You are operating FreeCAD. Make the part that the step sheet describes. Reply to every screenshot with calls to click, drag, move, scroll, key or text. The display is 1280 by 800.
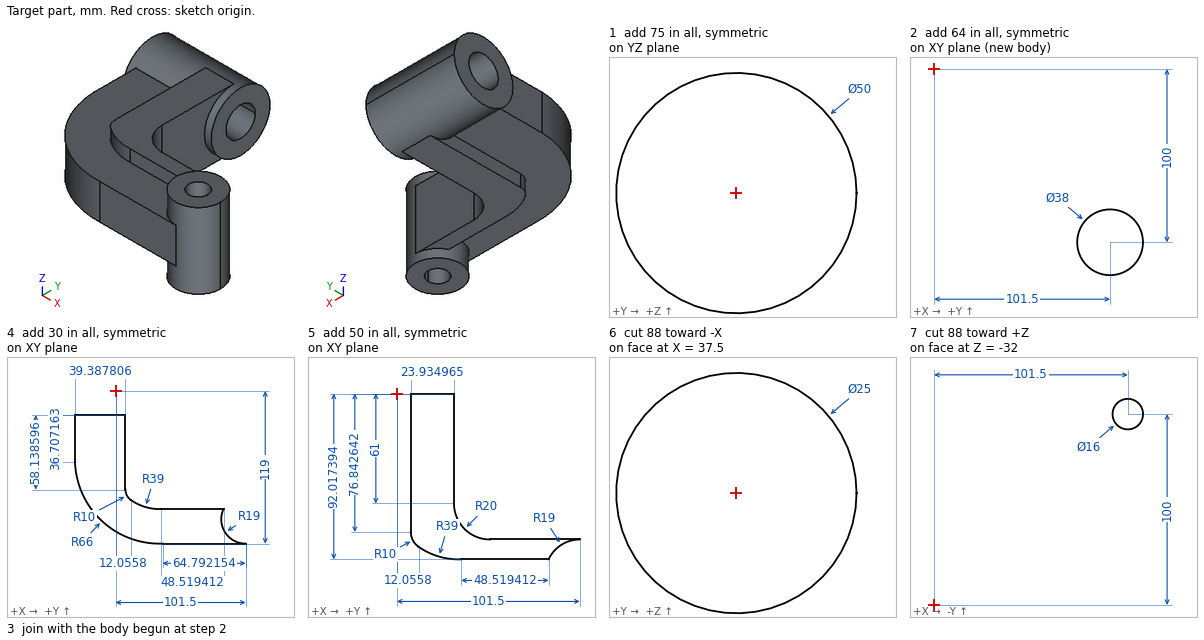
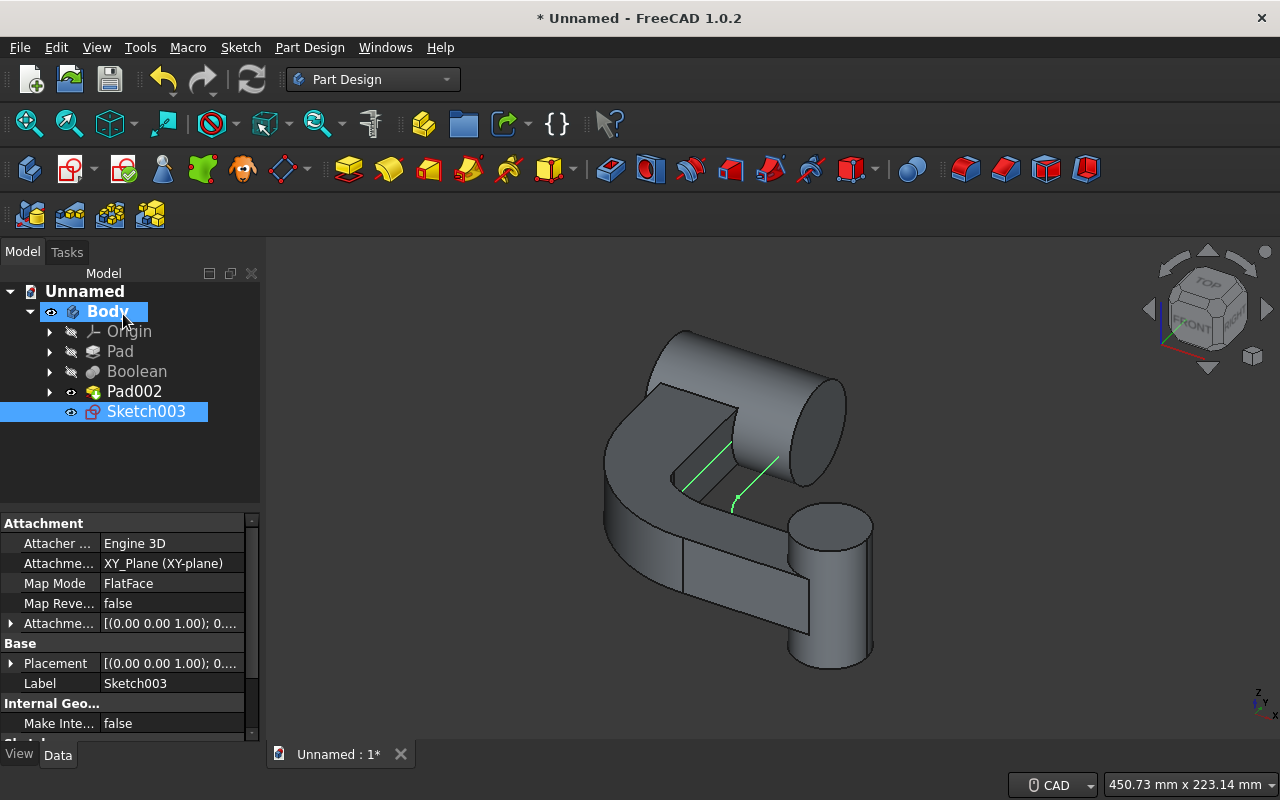
click(350, 170)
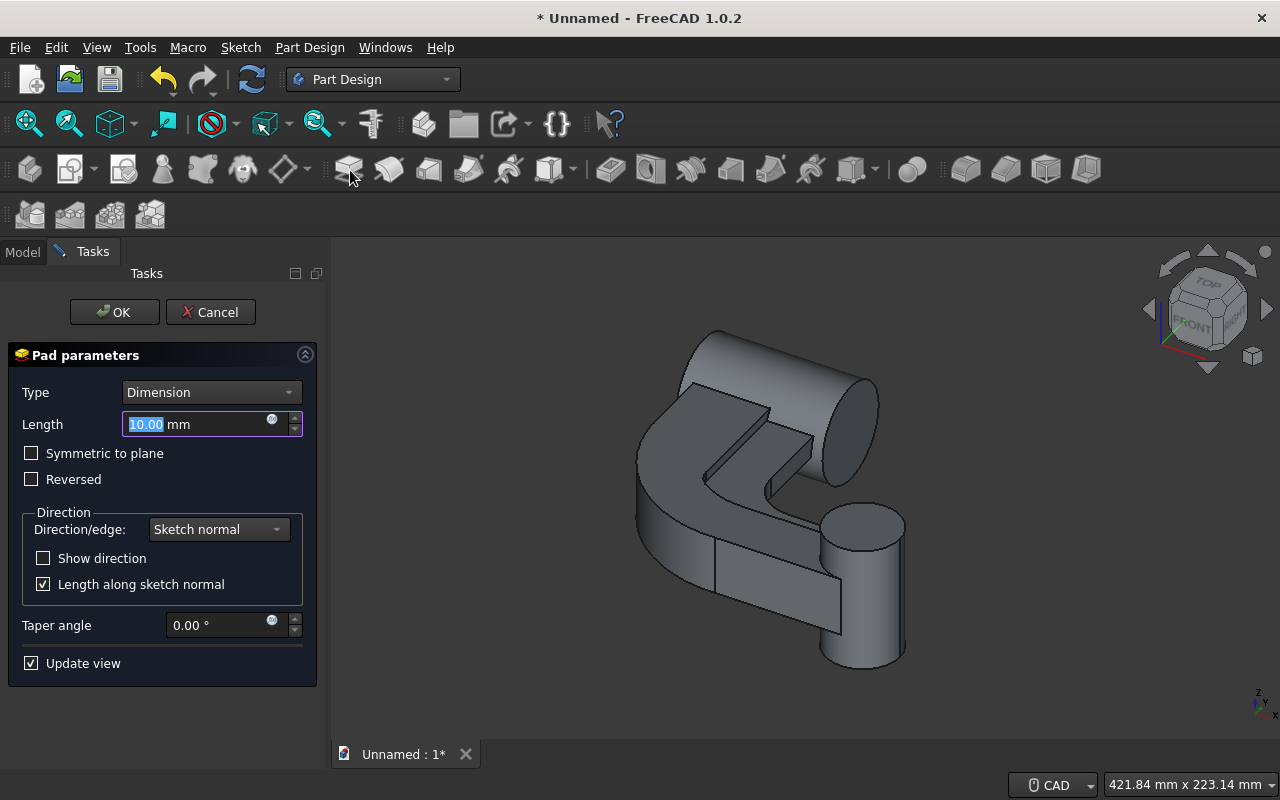
text(50)
key(Tab)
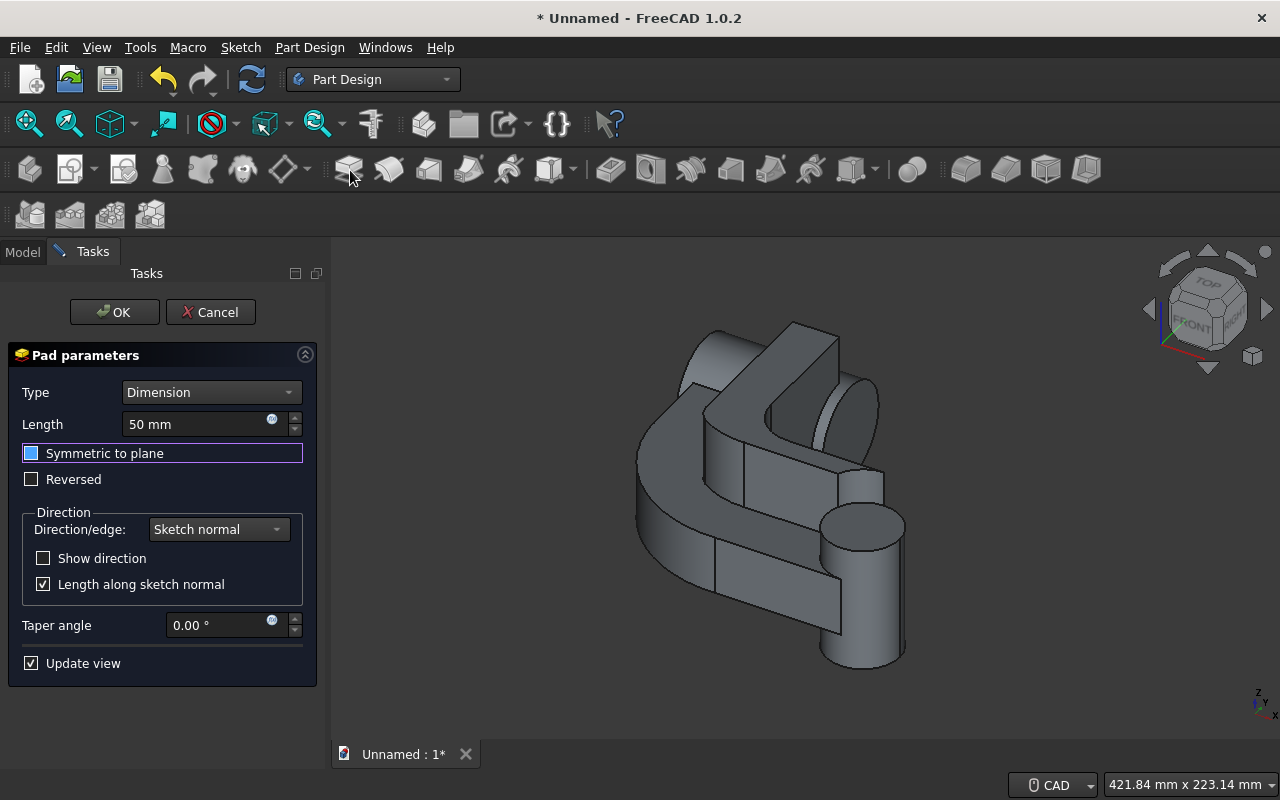
click(30, 453)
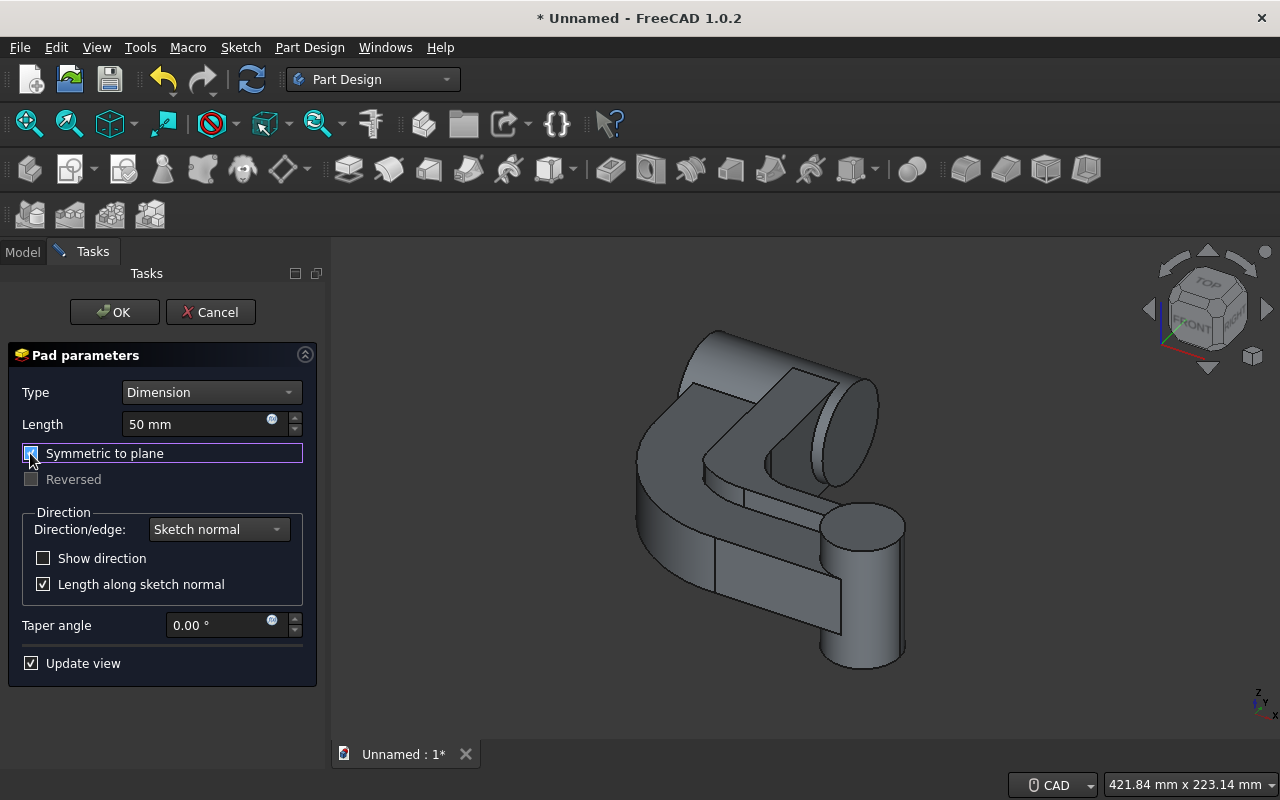
click(115, 312)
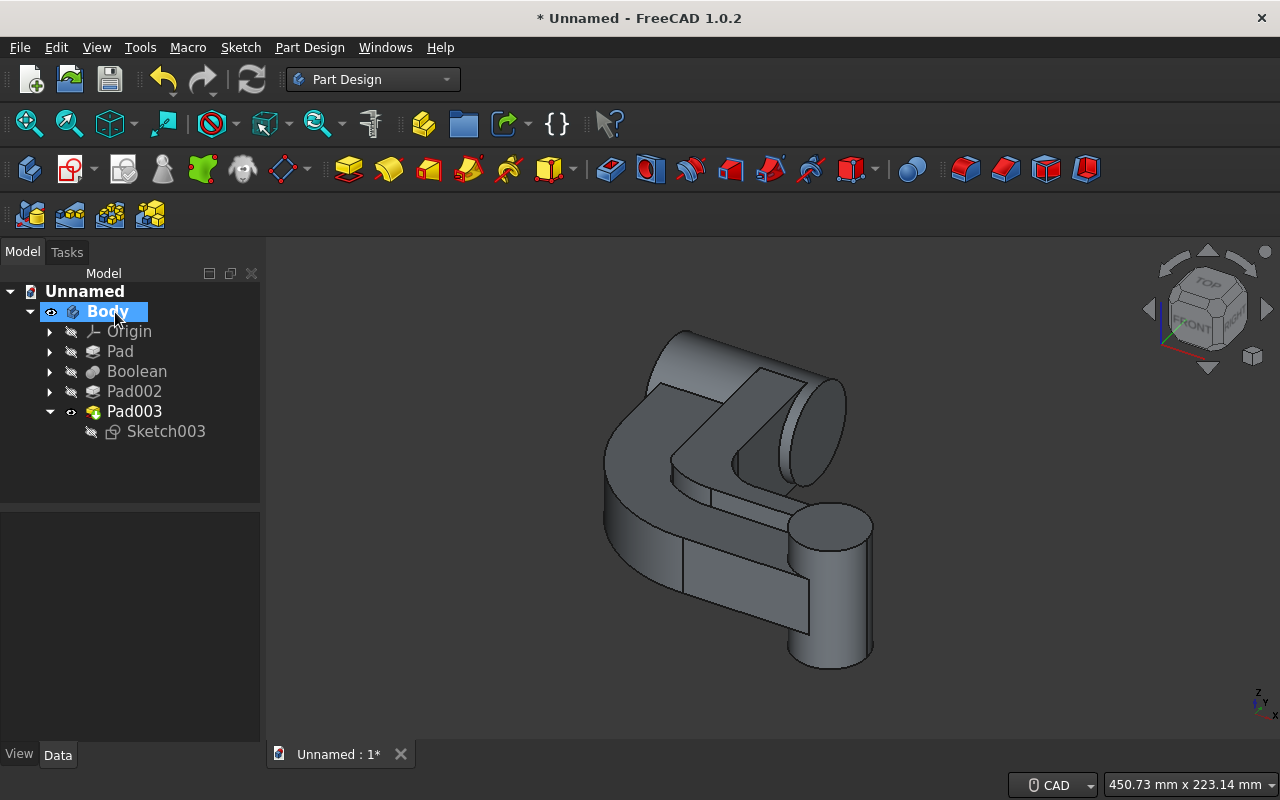
click(818, 432)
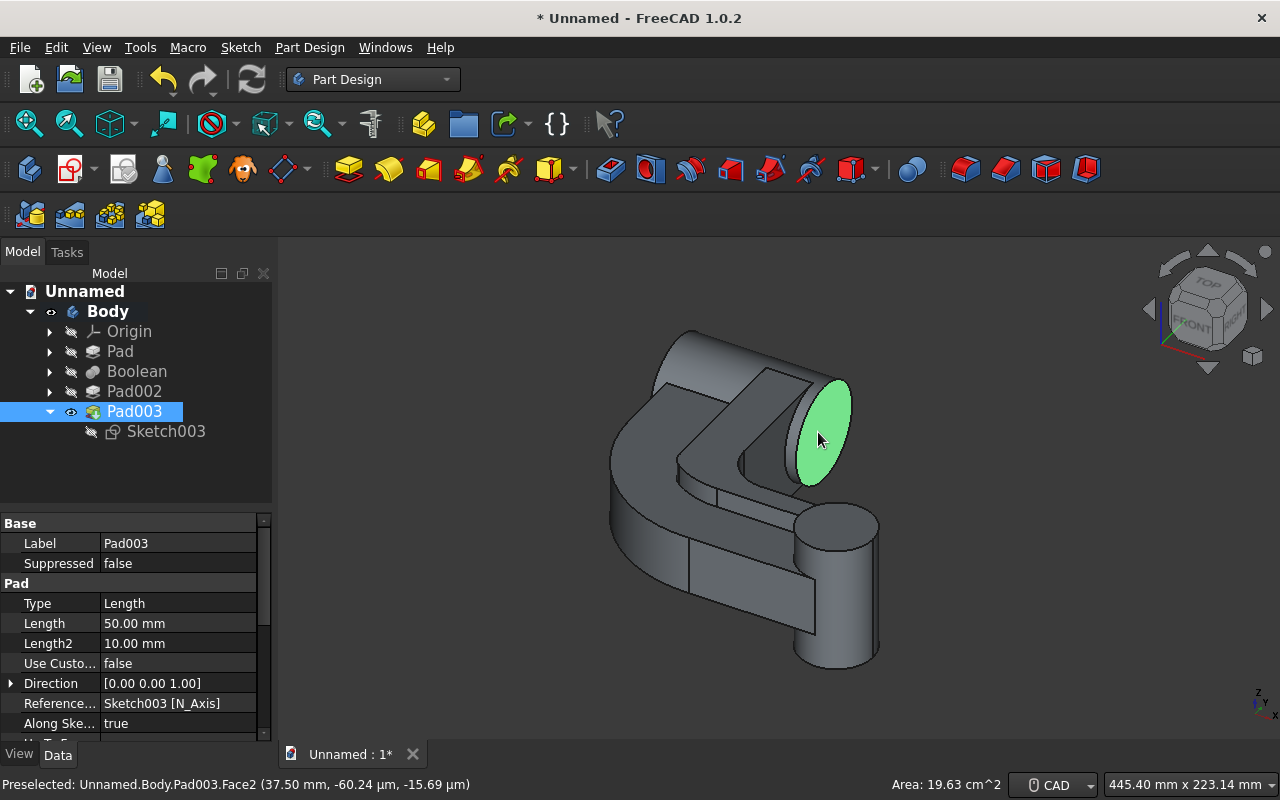
click(70, 170)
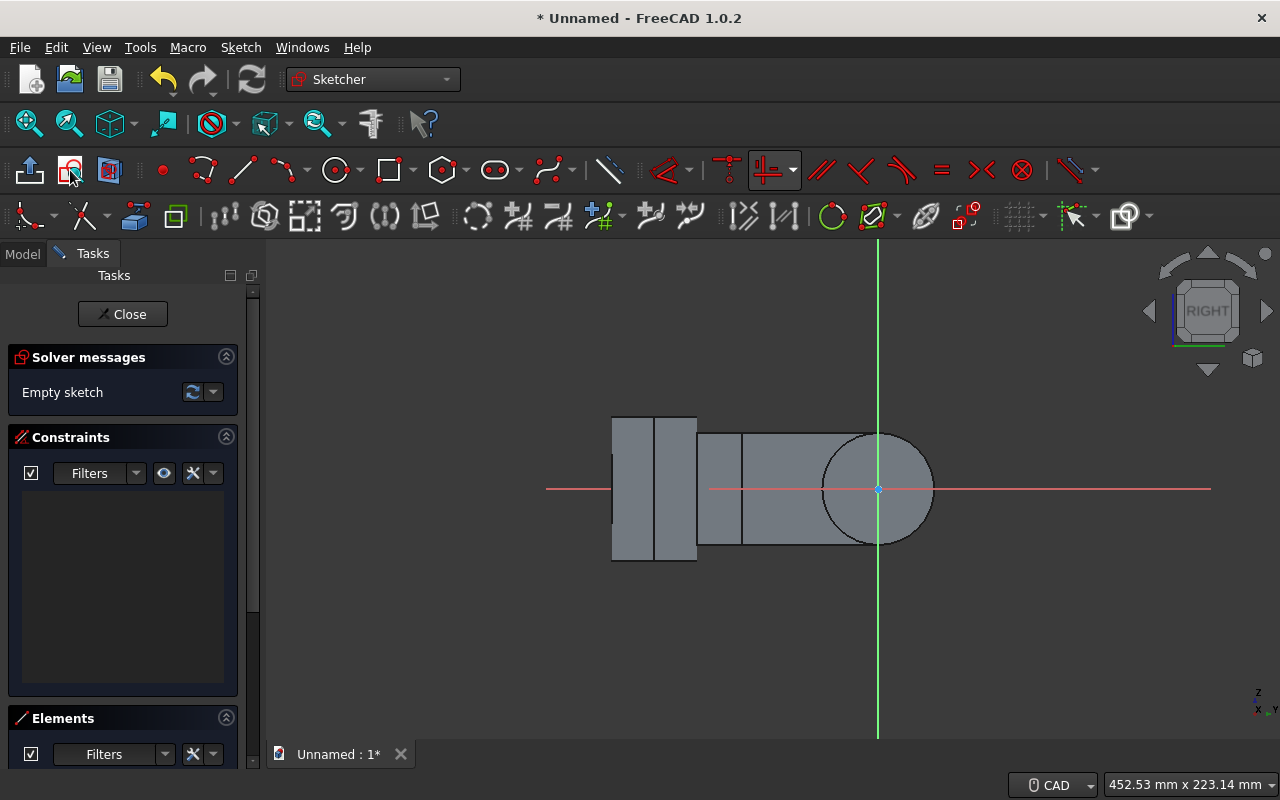
key(q)
key(s)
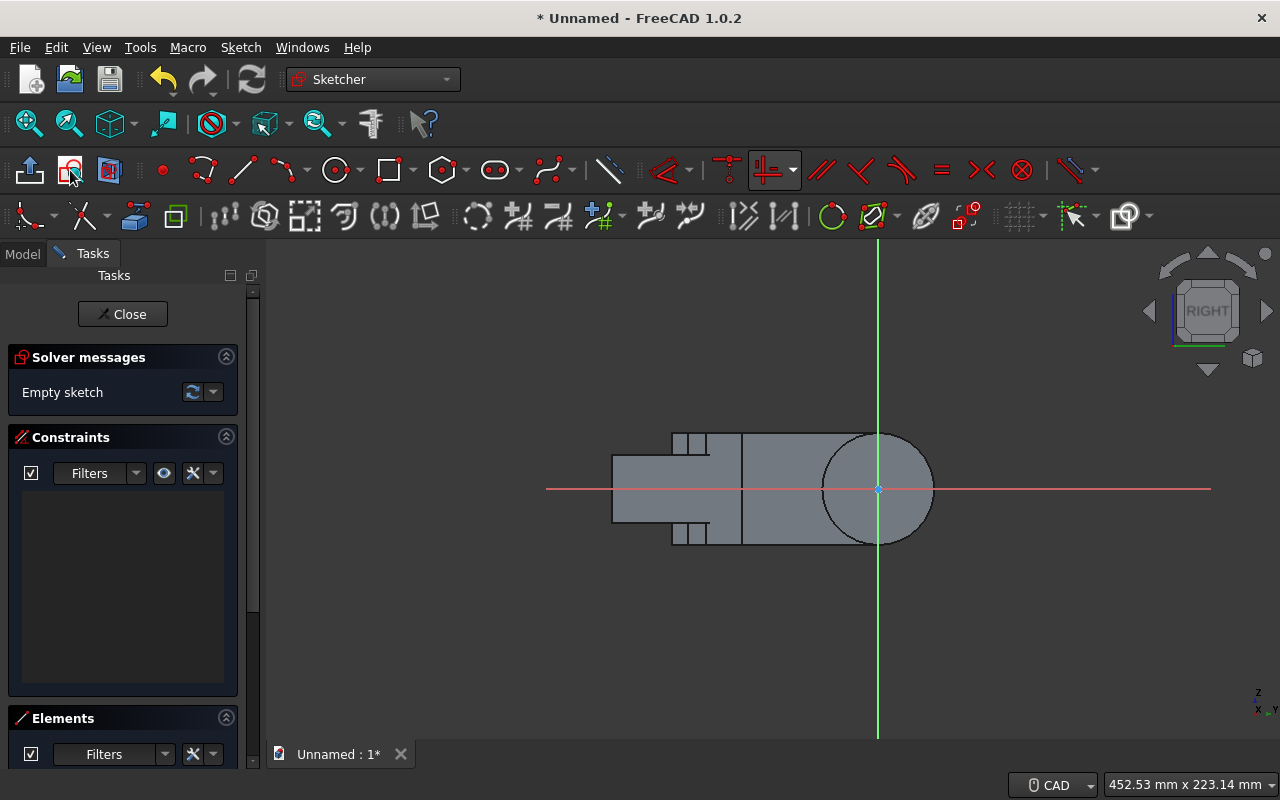
scroll(913, 489, up, 9)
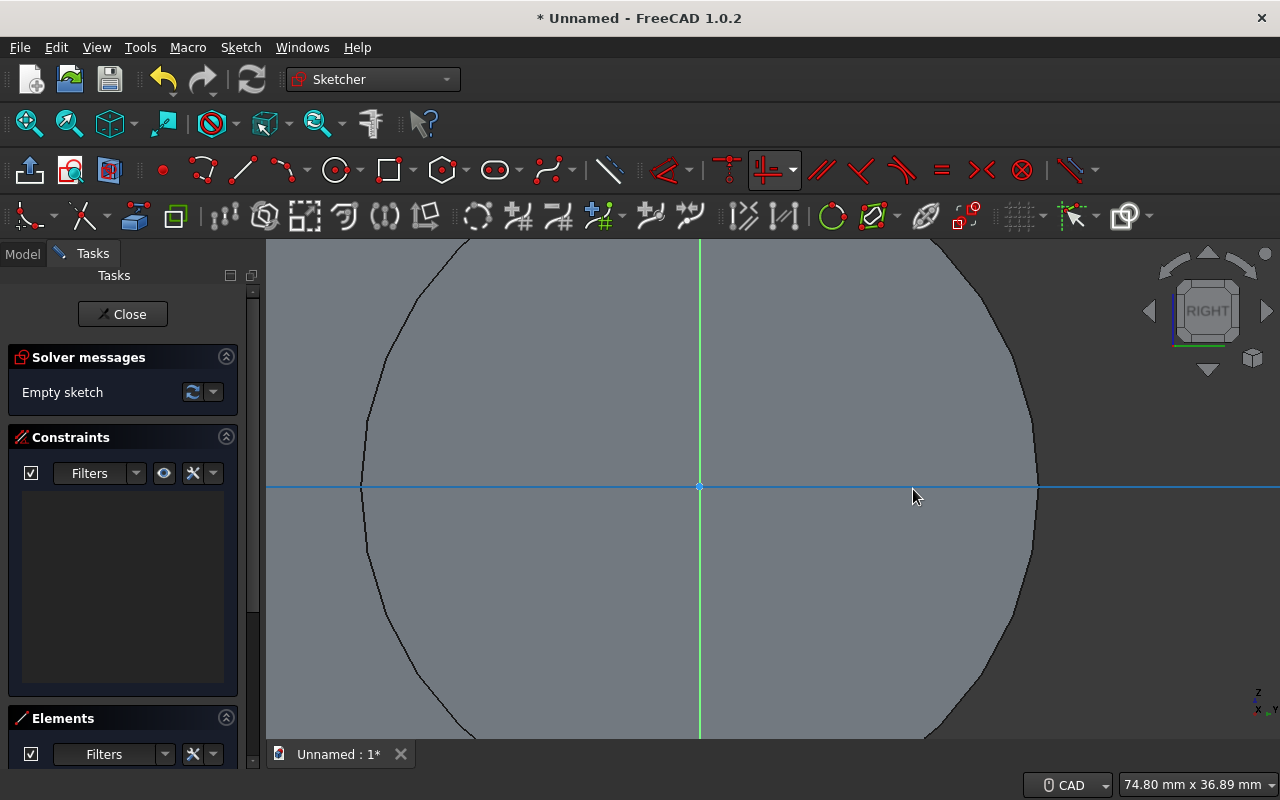
key(g)
key(c)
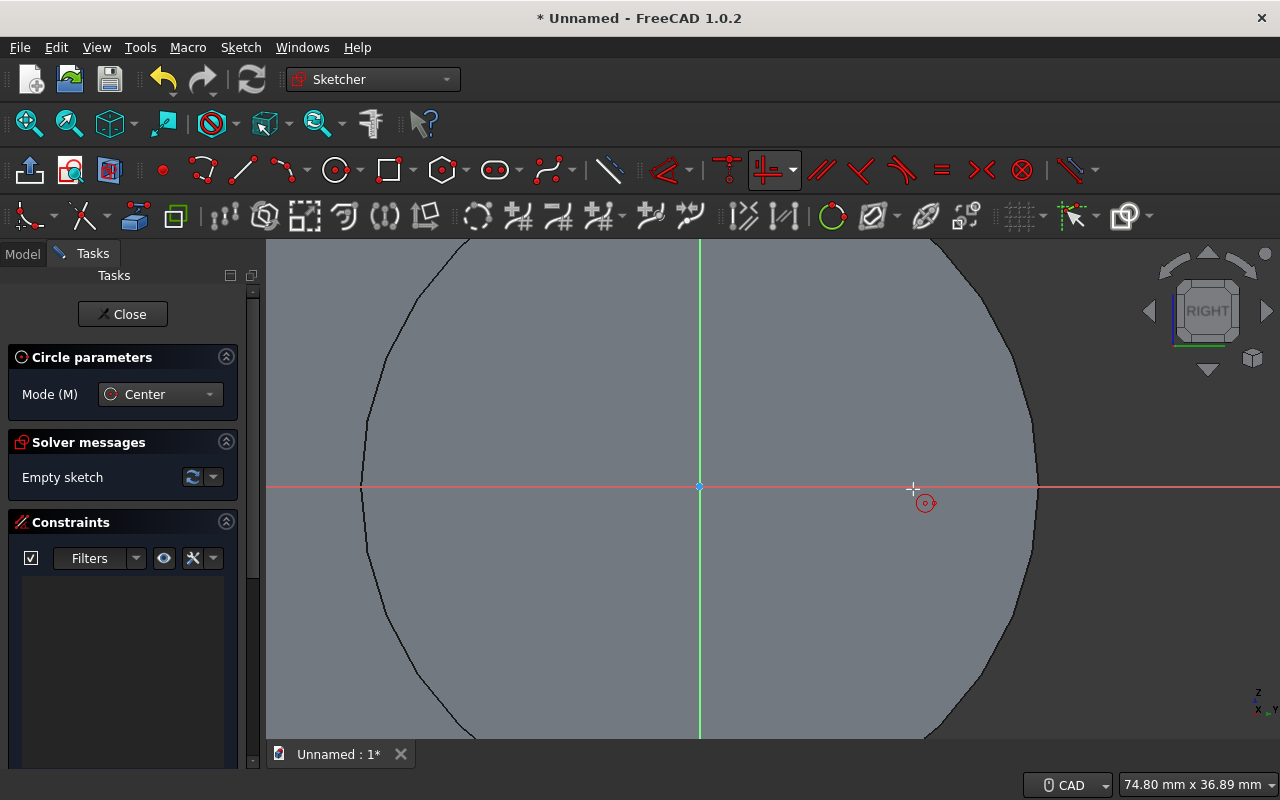
click(700, 487)
click(820, 367)
key(Escape)